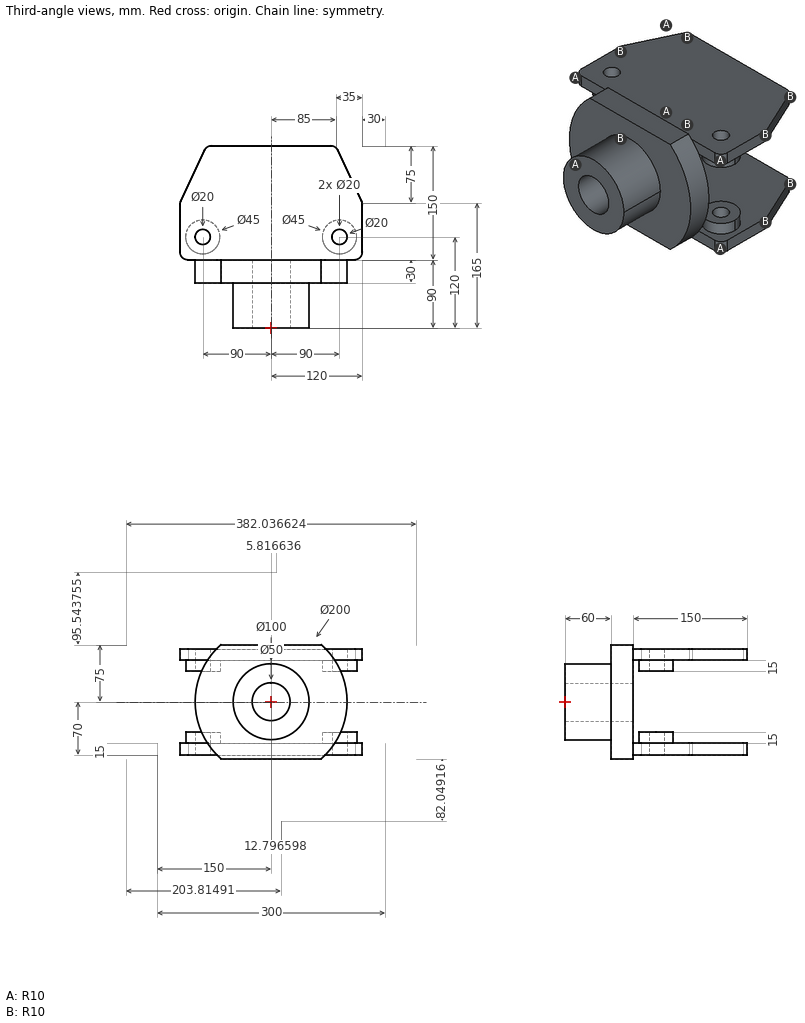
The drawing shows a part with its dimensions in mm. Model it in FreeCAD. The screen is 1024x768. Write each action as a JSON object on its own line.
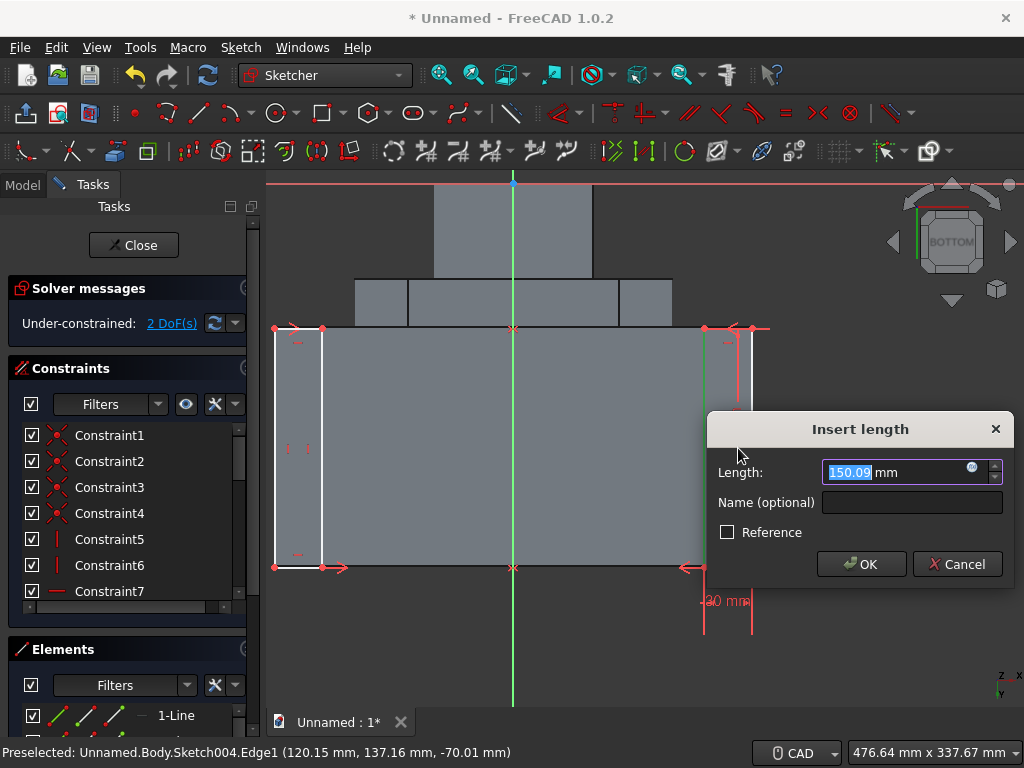
{"action": "type", "text": "150"}
{"action": "key", "text": "Return"}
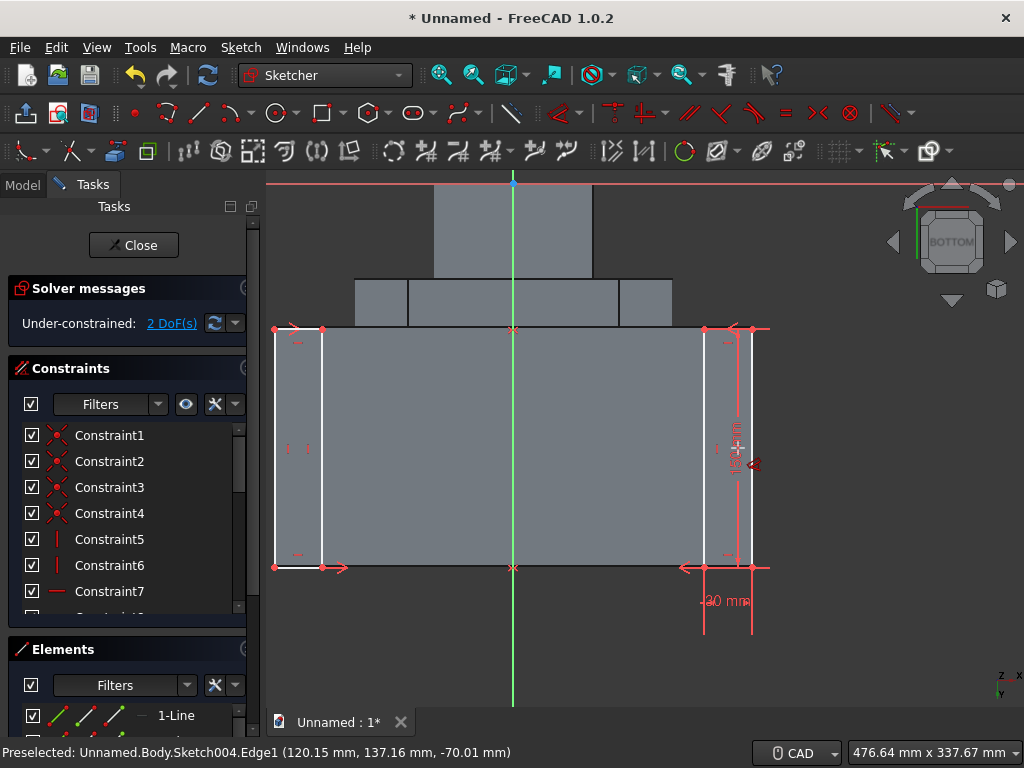
{"action": "left_click", "coordinate": [704, 329]}
{"action": "left_click", "coordinate": [738, 264]}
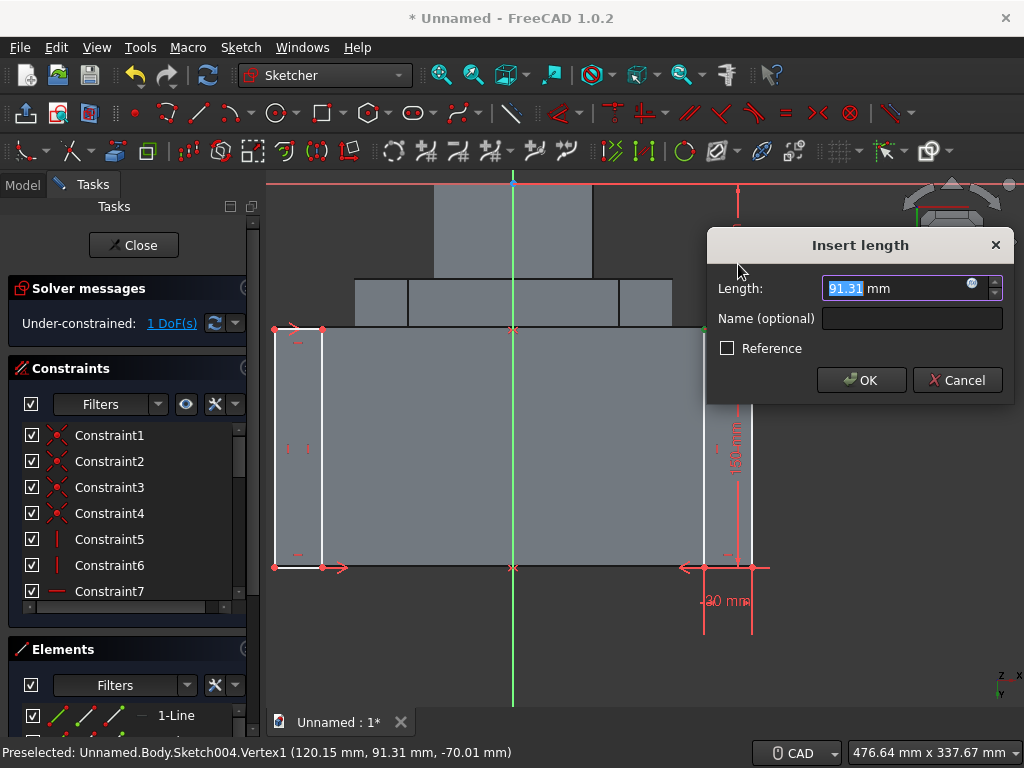
{"action": "type", "text": "90"}
{"action": "key", "text": "Return"}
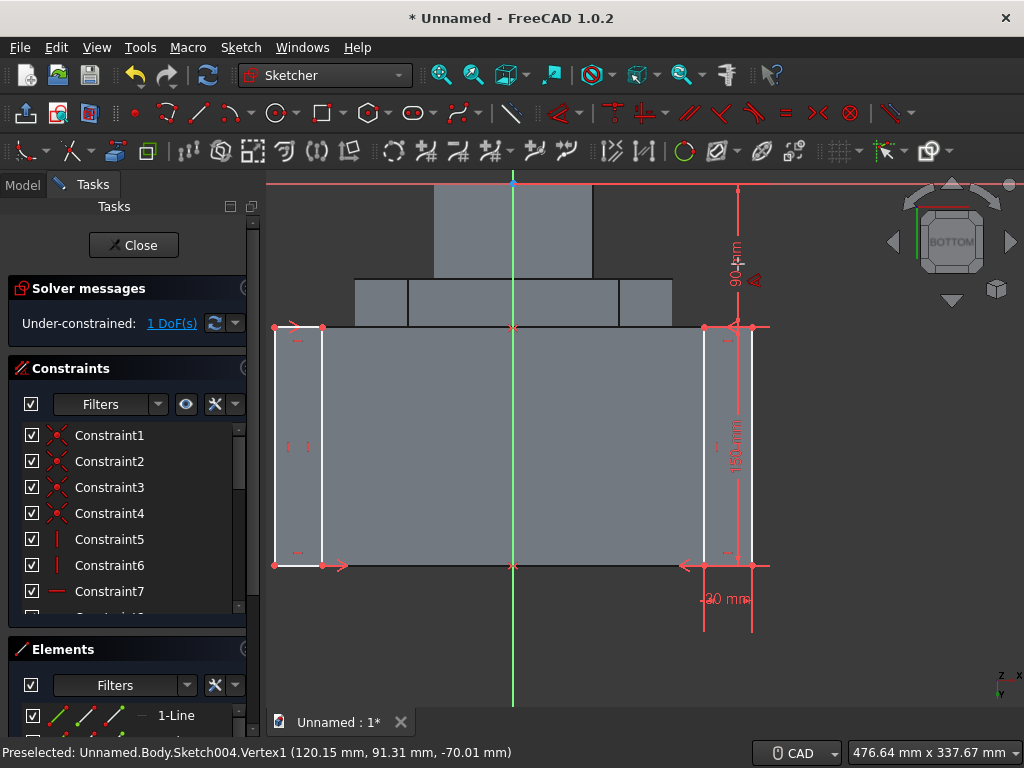
{"action": "left_click", "coordinate": [704, 327]}
{"action": "left_click", "coordinate": [609, 361]}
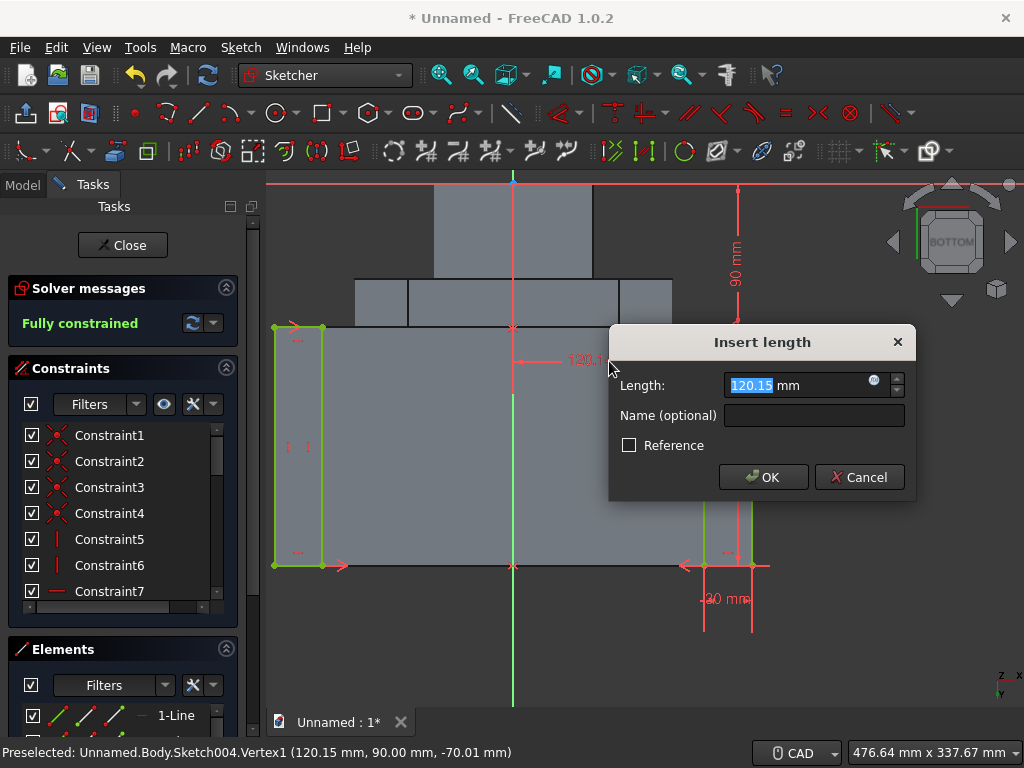
{"action": "type", "text": "120"}
{"action": "key", "text": "Return"}
{"action": "key", "text": "Escape"}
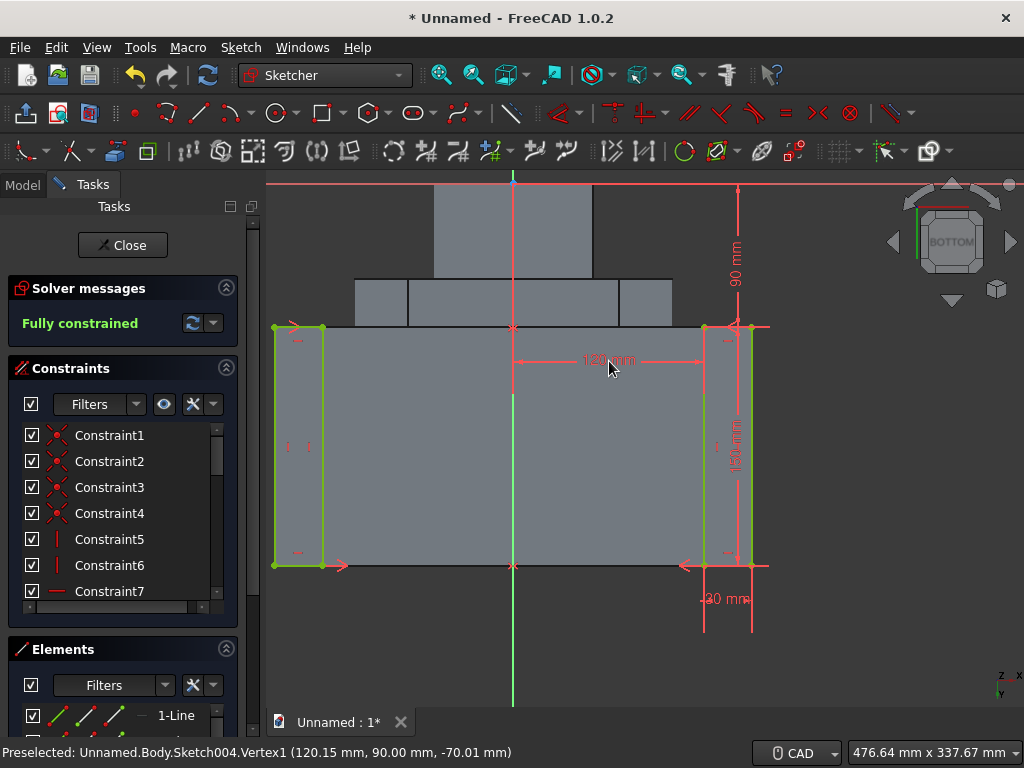
{"action": "left_click", "coordinate": [123, 245]}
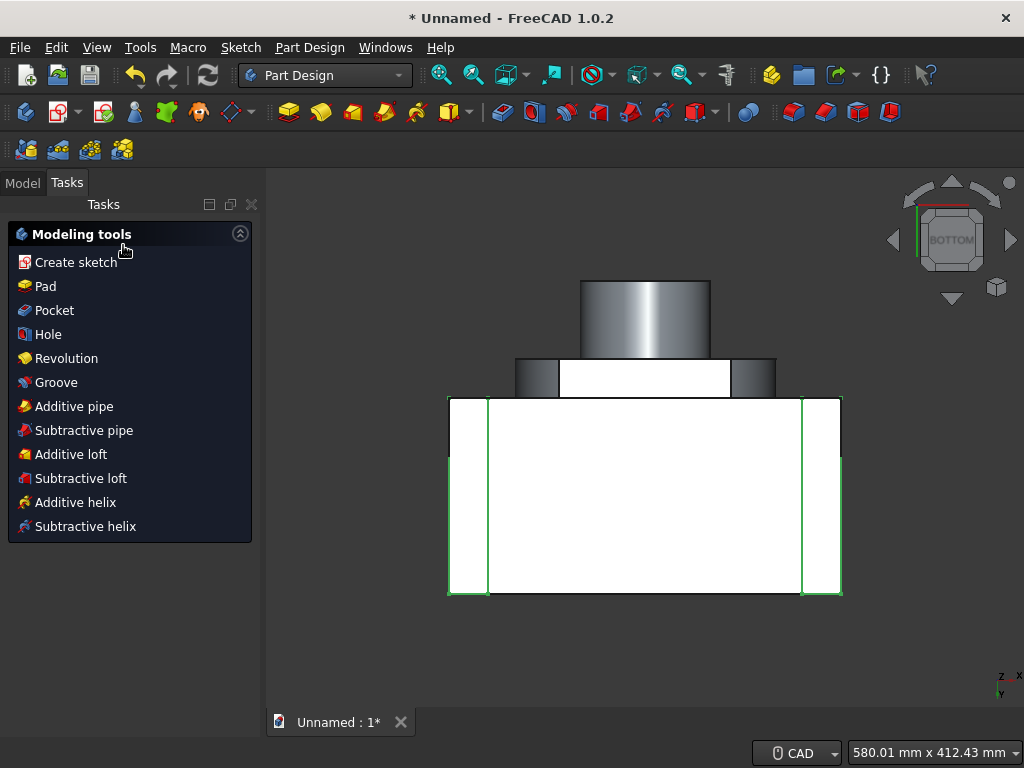
{"action": "left_click", "coordinate": [504, 112]}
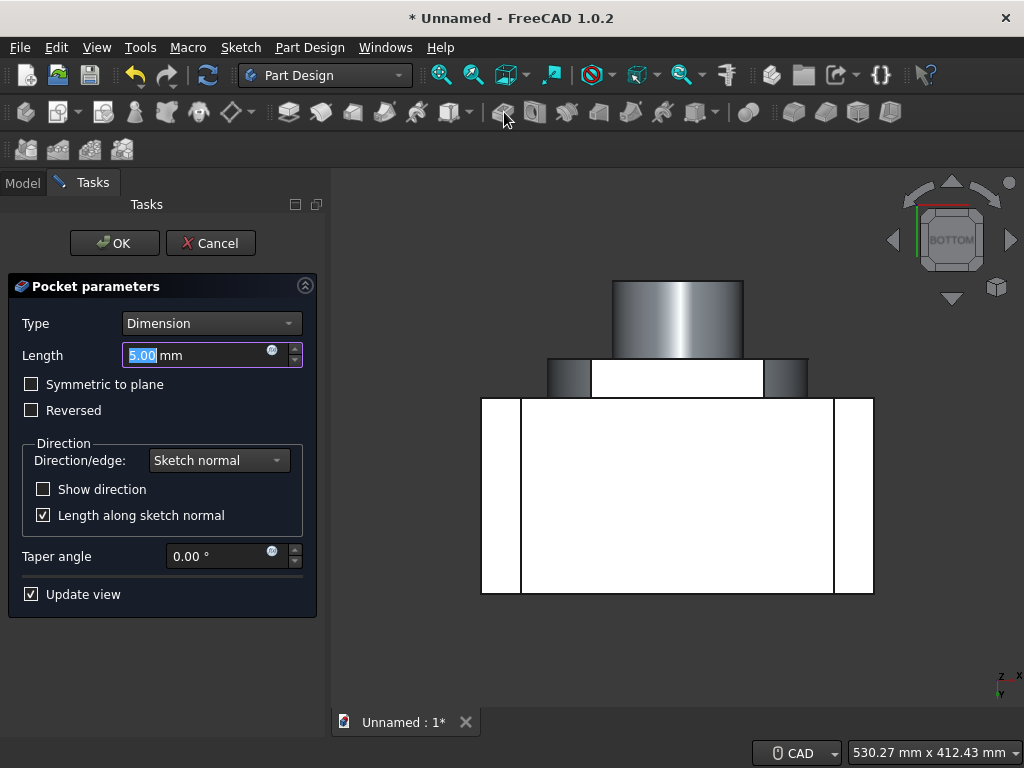
{"action": "left_click", "coordinate": [212, 324]}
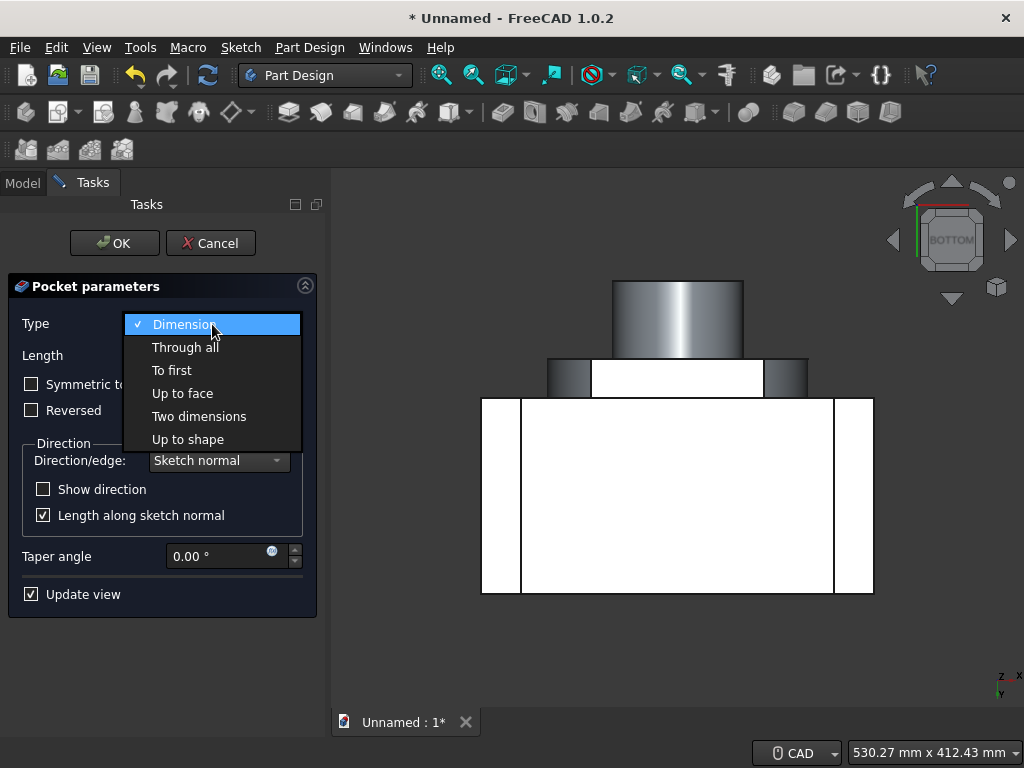
{"action": "left_click", "coordinate": [212, 348]}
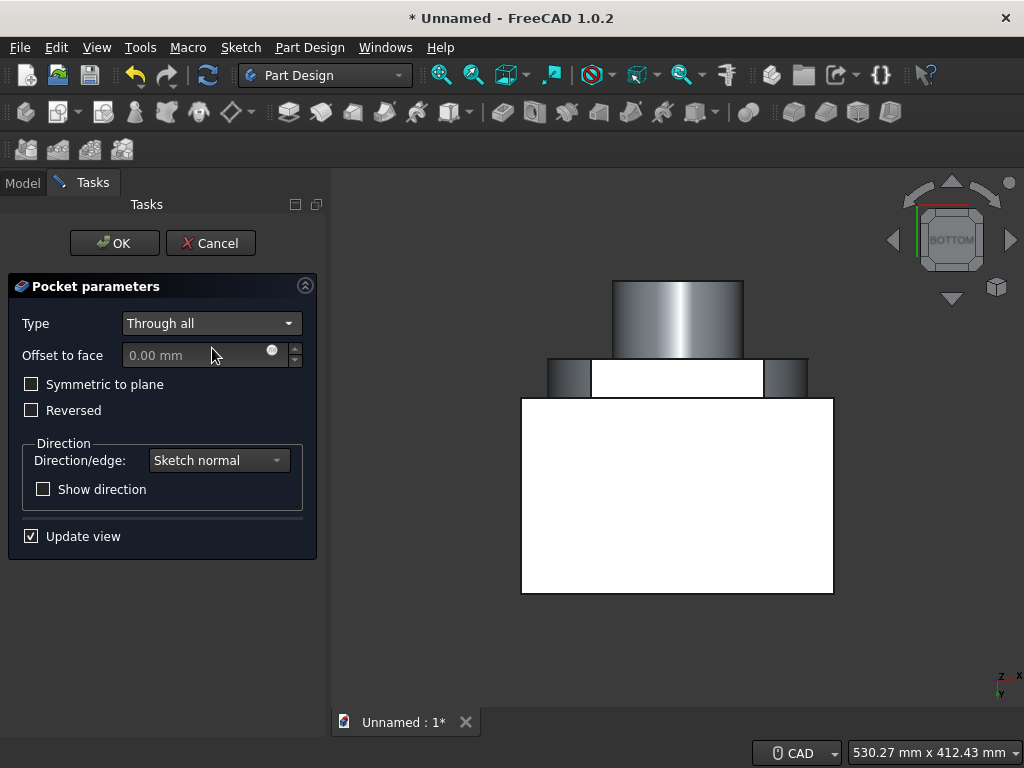
{"action": "left_click", "coordinate": [115, 243]}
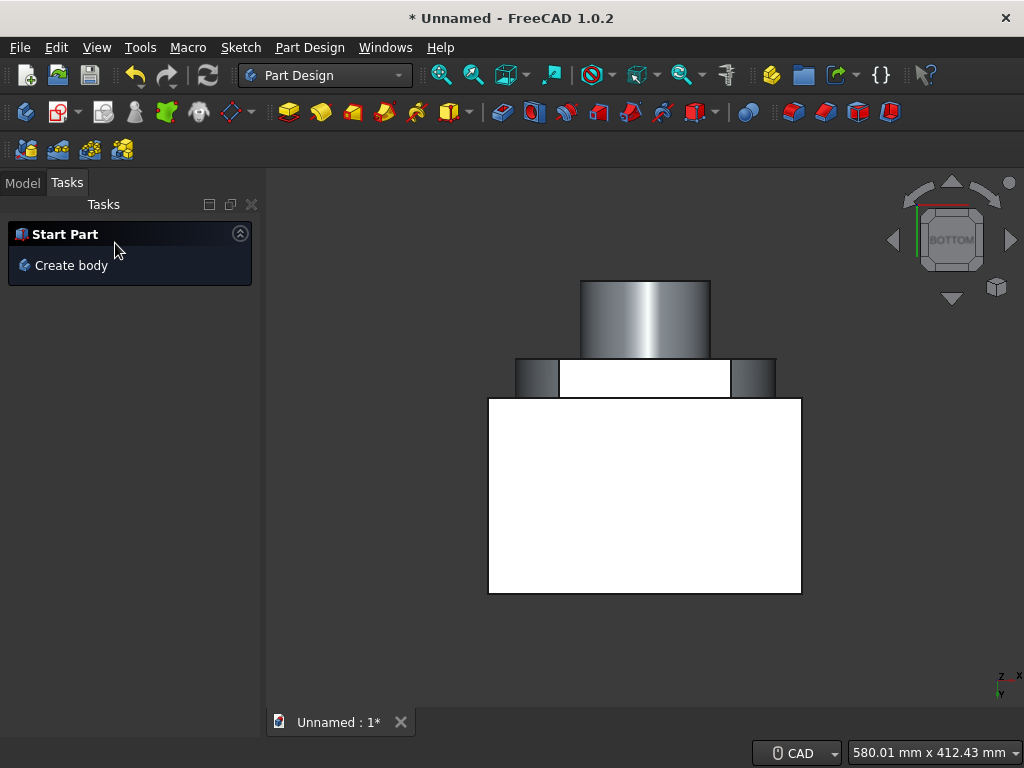
{"action": "scroll", "coordinate": [488, 593], "scroll_direction": "up", "scroll_amount": 4}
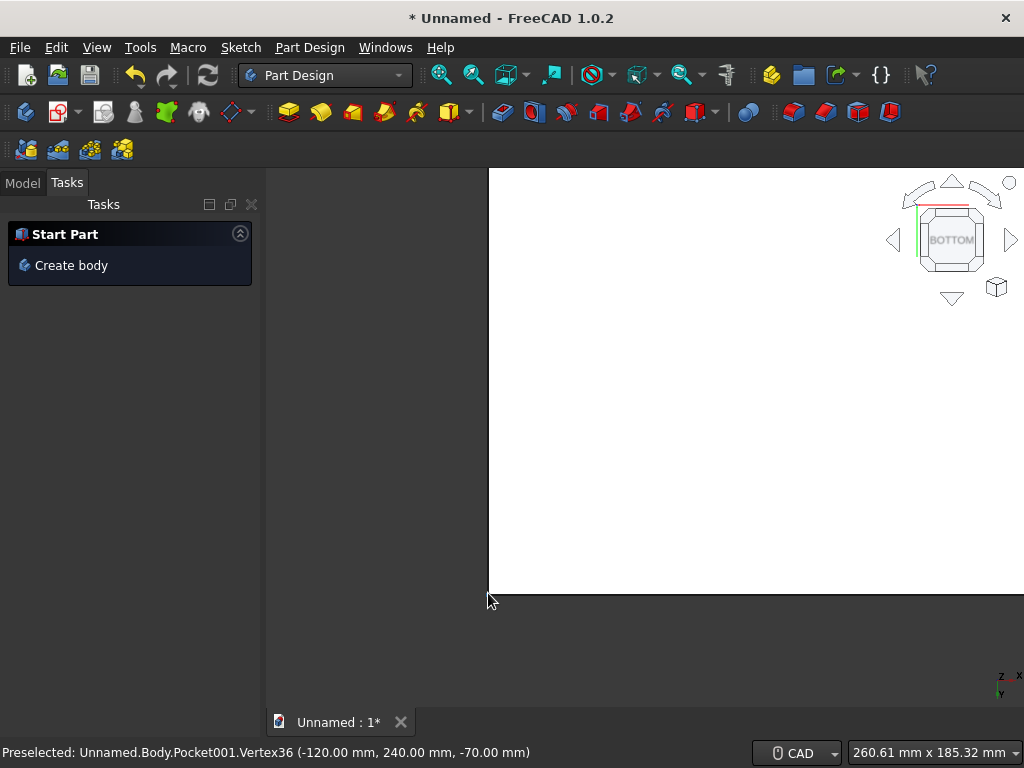
{"action": "left_click", "coordinate": [442, 76]}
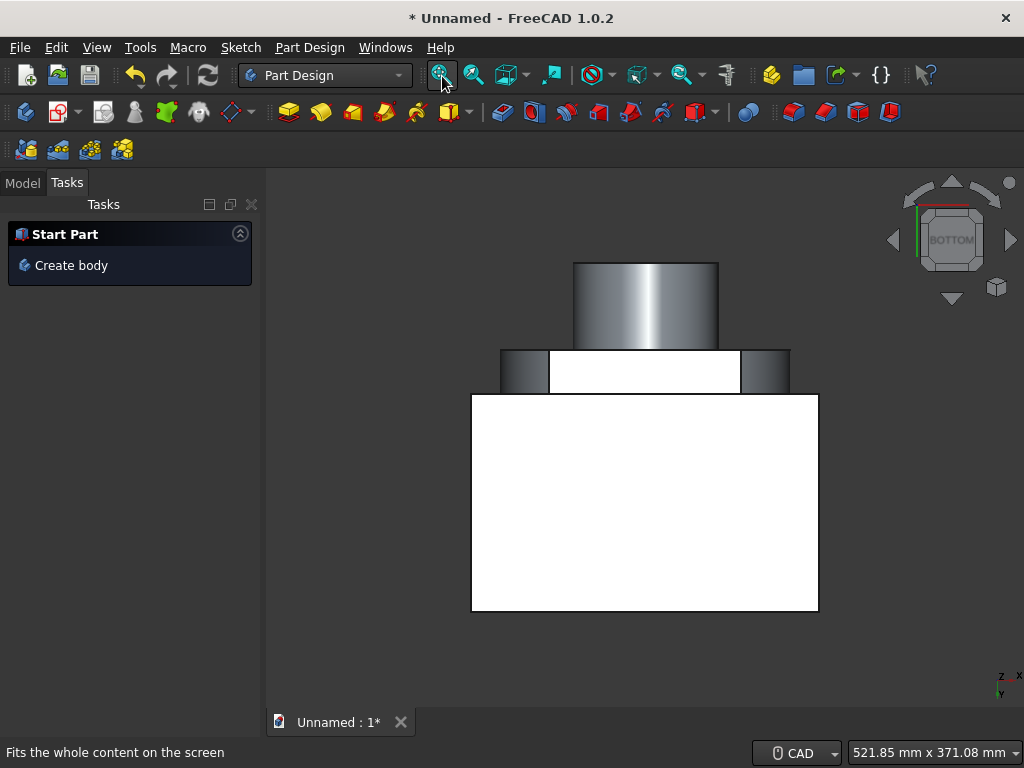
{"action": "key", "text": "0"}